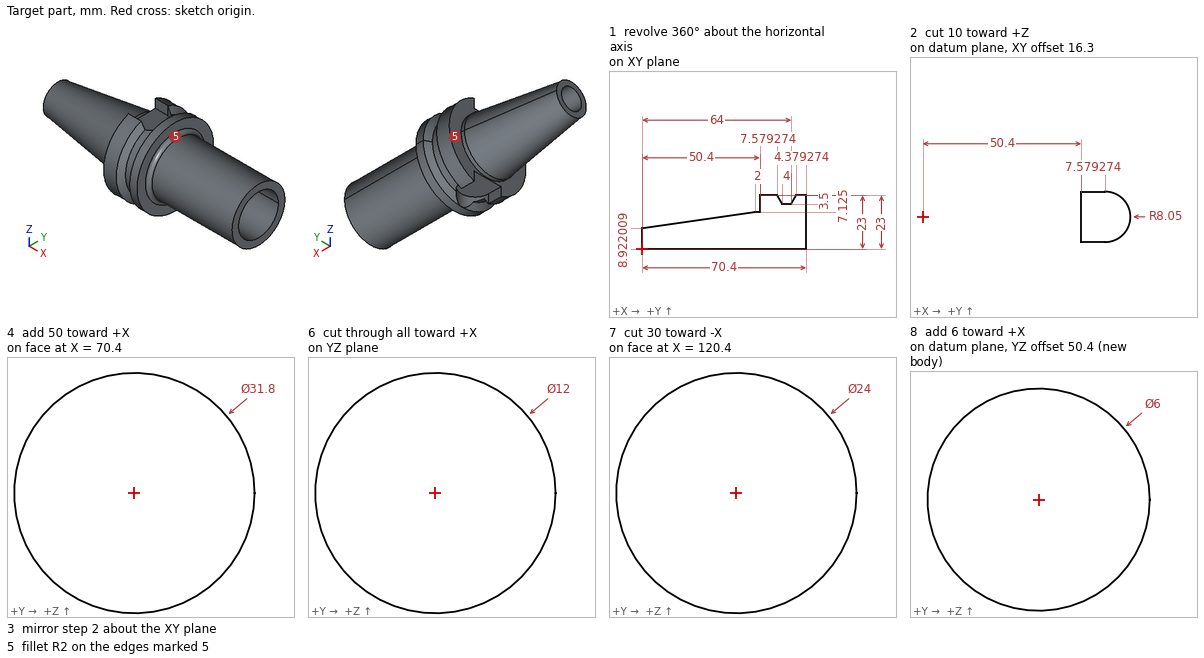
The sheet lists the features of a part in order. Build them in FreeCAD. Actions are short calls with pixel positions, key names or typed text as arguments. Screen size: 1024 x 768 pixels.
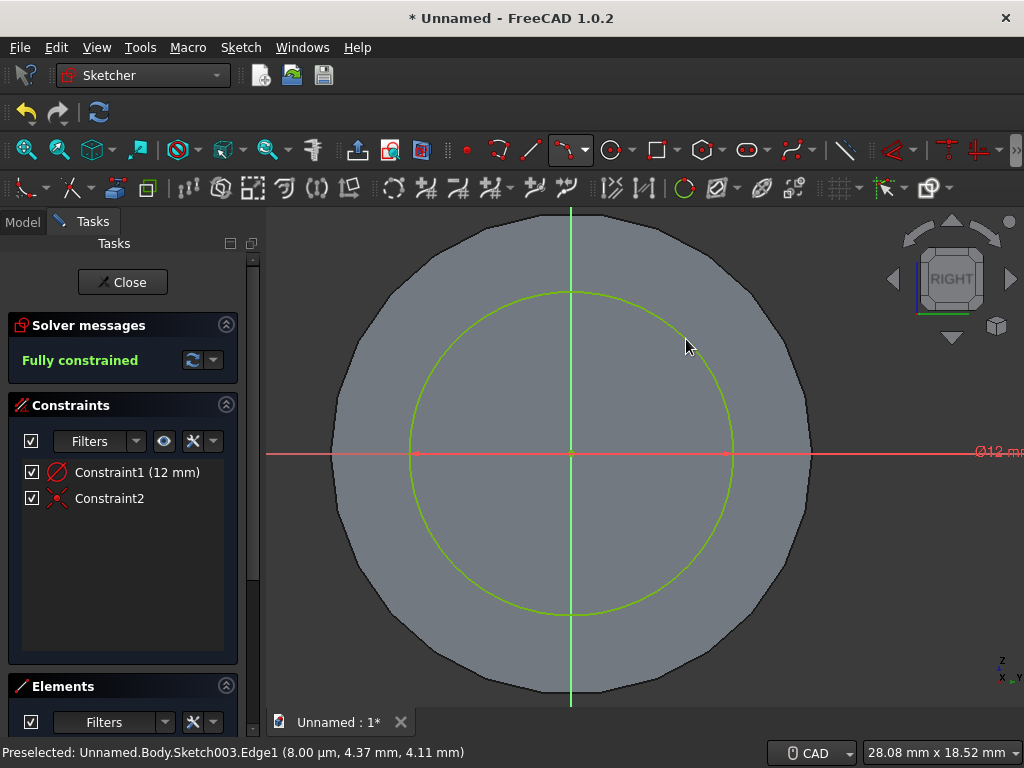
click(123, 282)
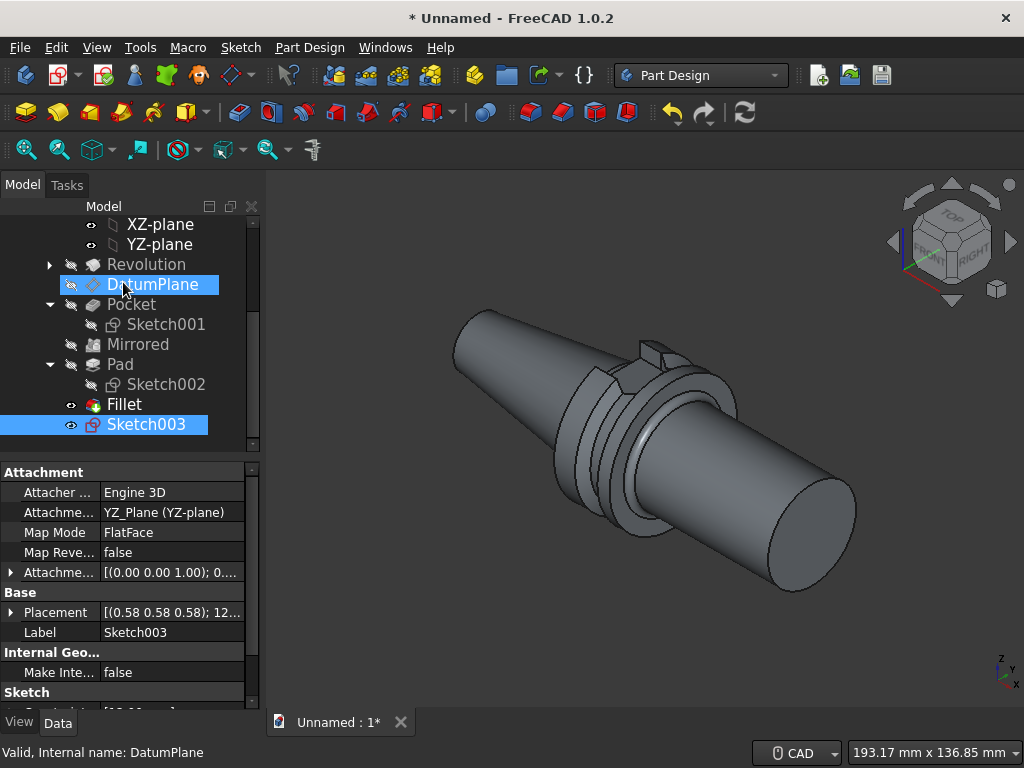
click(240, 112)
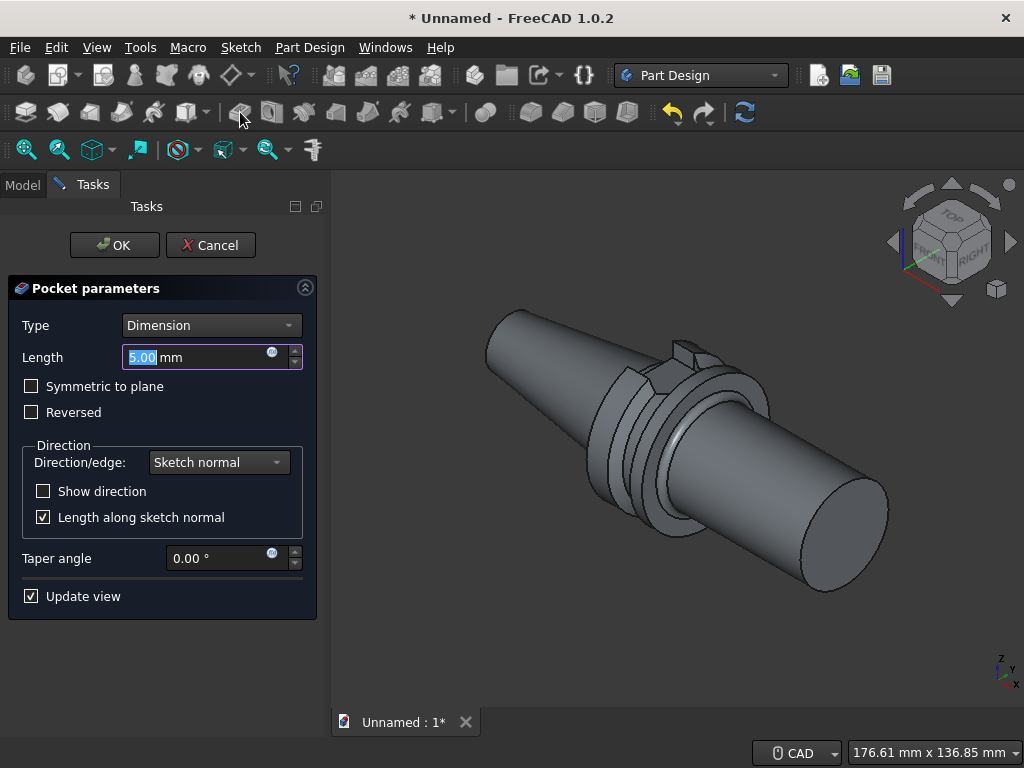
click(212, 326)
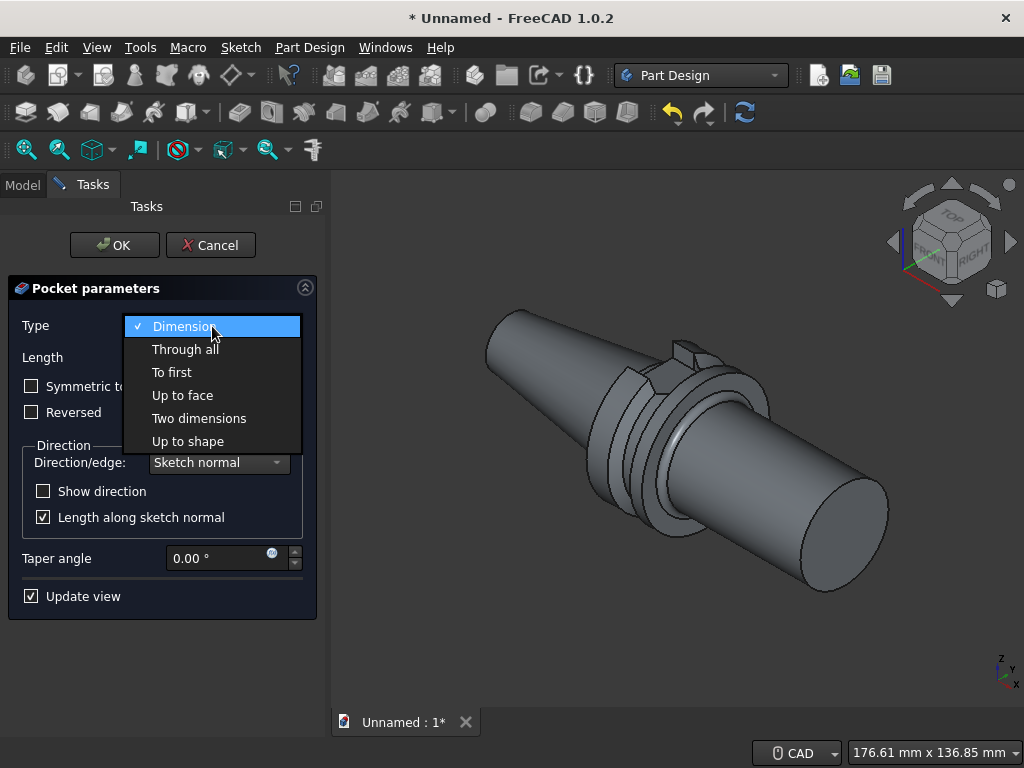
click(212, 350)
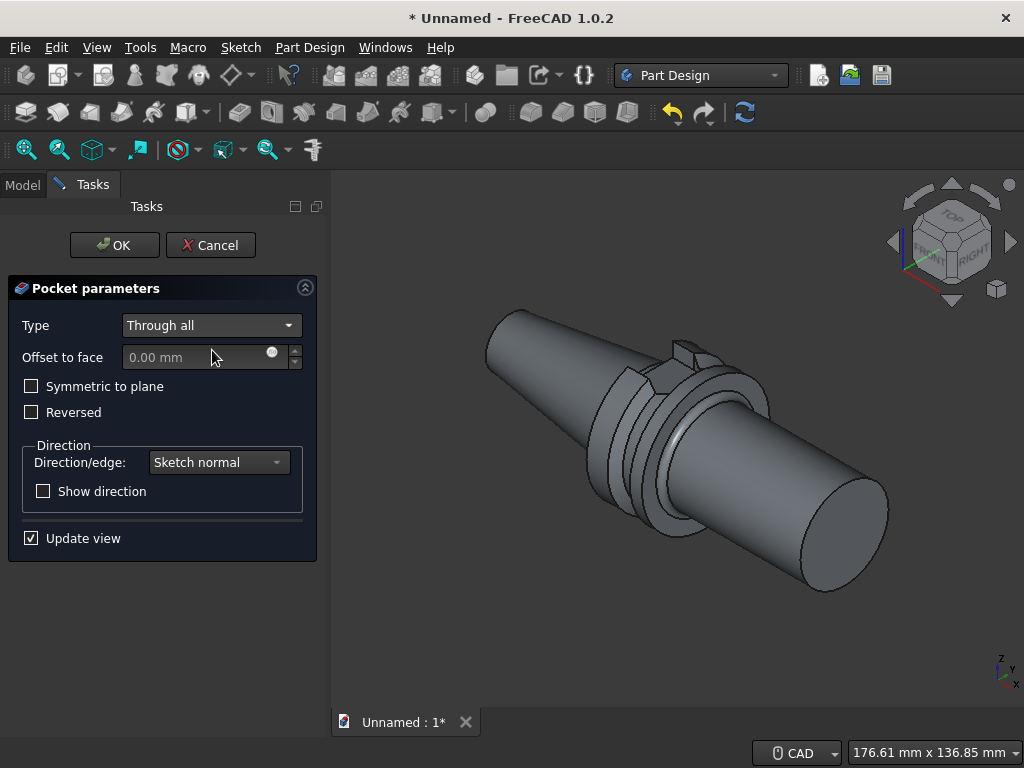
click(30, 412)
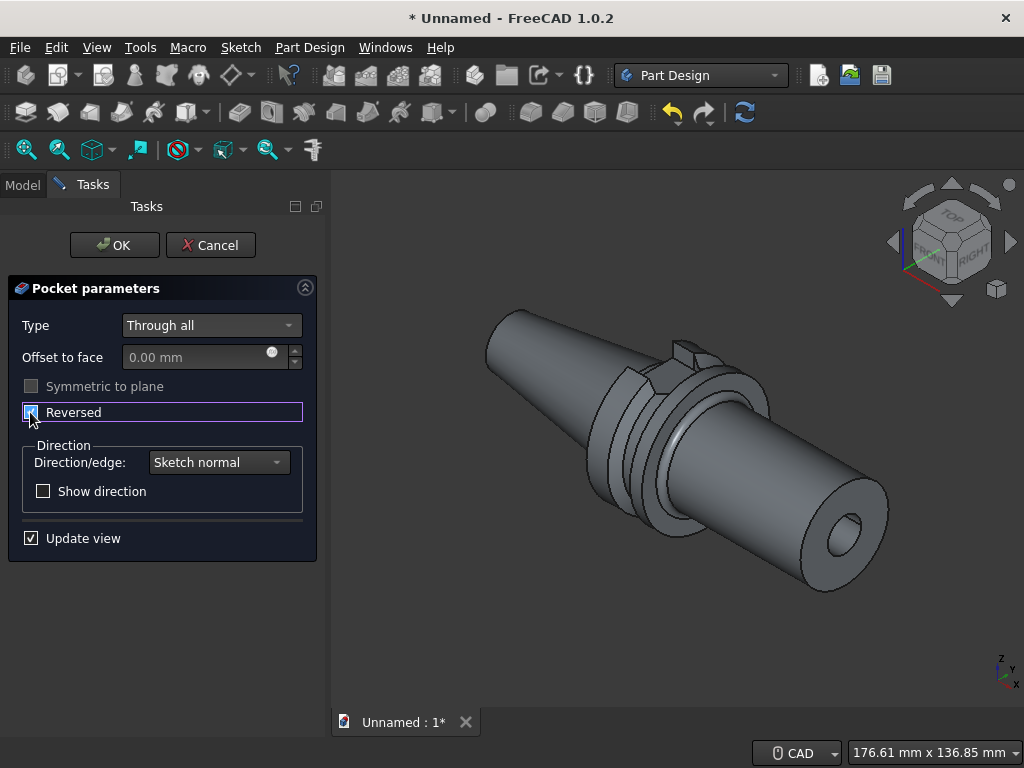
click(115, 245)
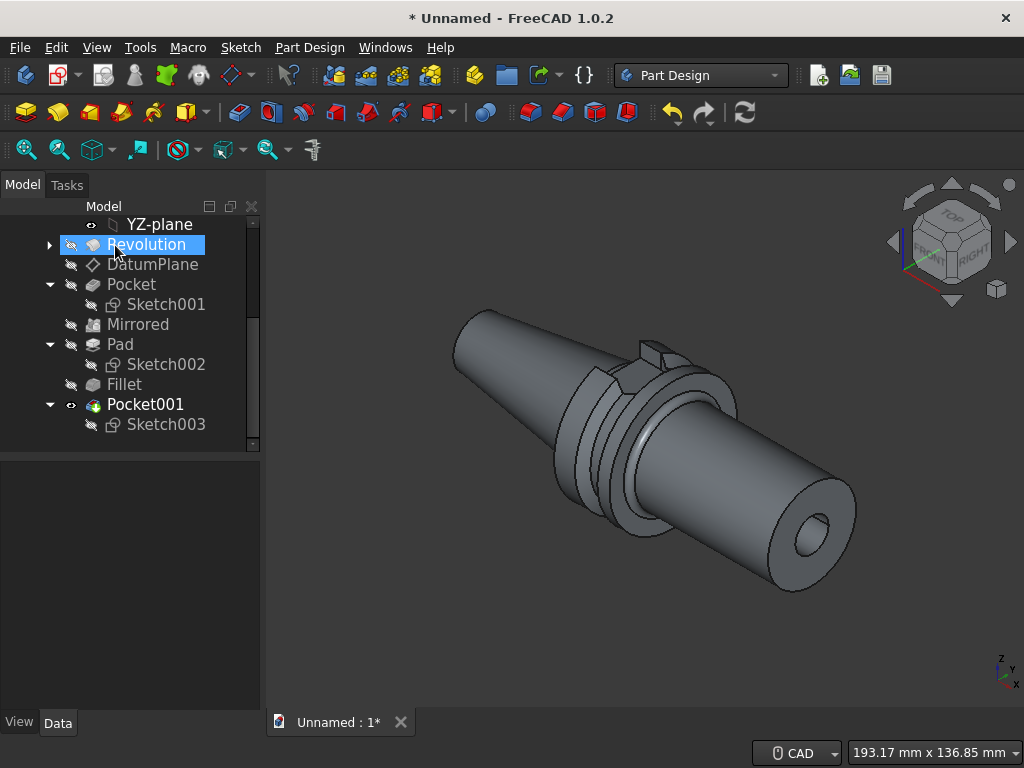
click(825, 498)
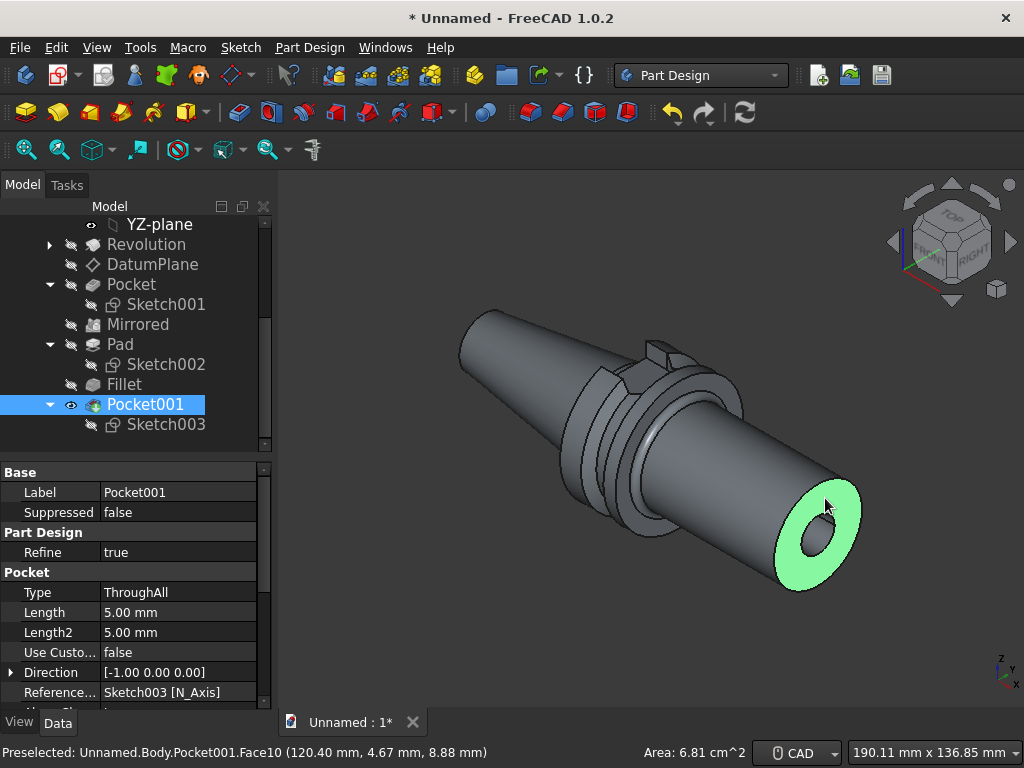
click(58, 76)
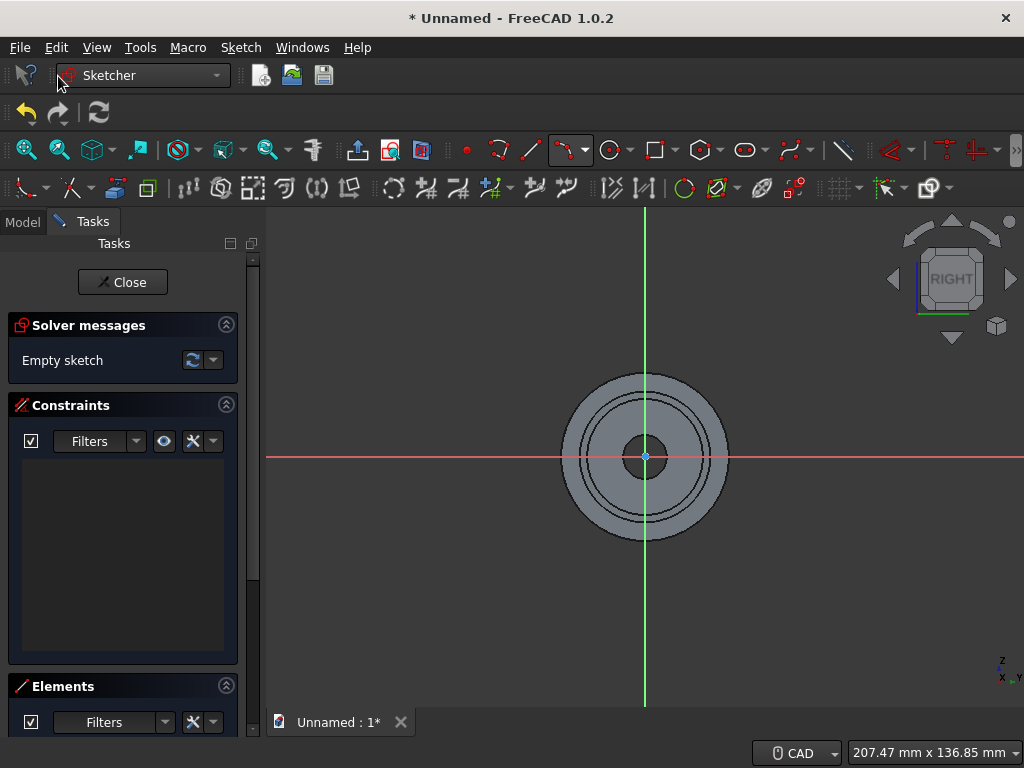
scroll(675, 457, up, 6)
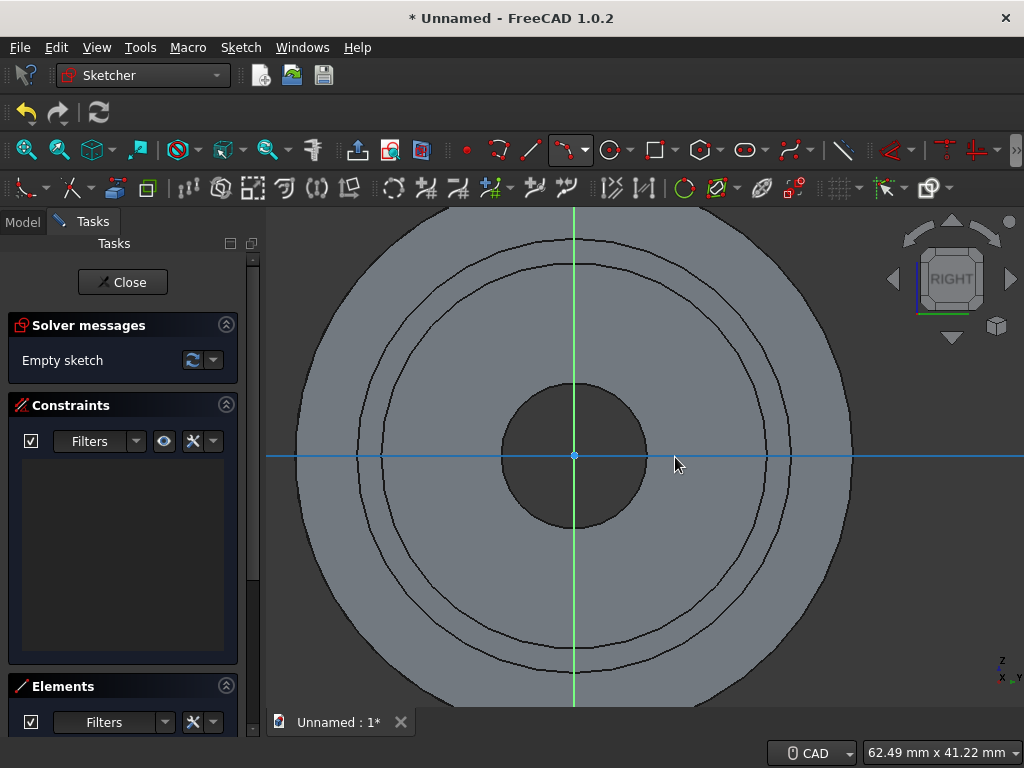
key(g)
key(c)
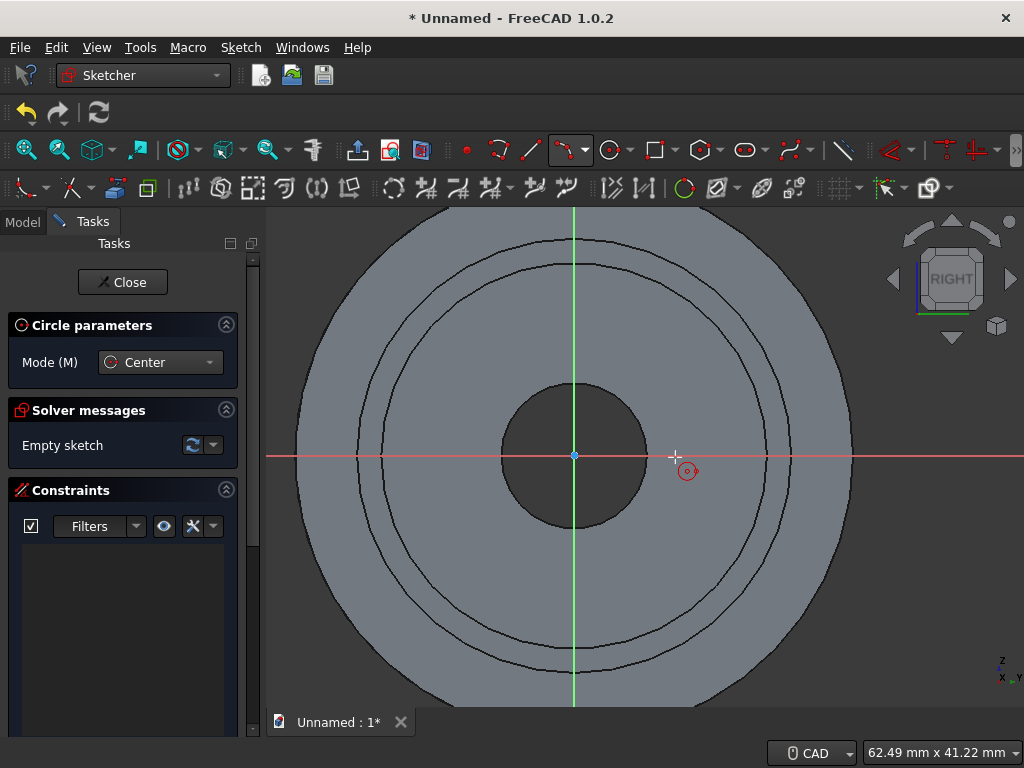
click(574, 456)
move(677, 353)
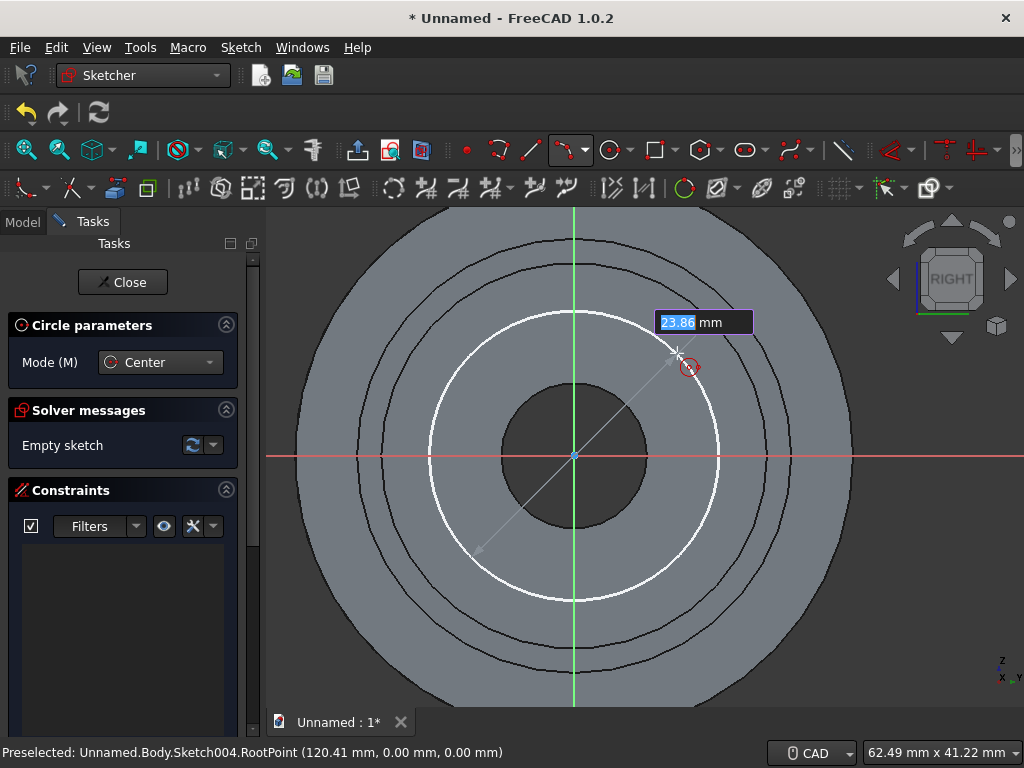
text(24)
key(Return)
key(Escape)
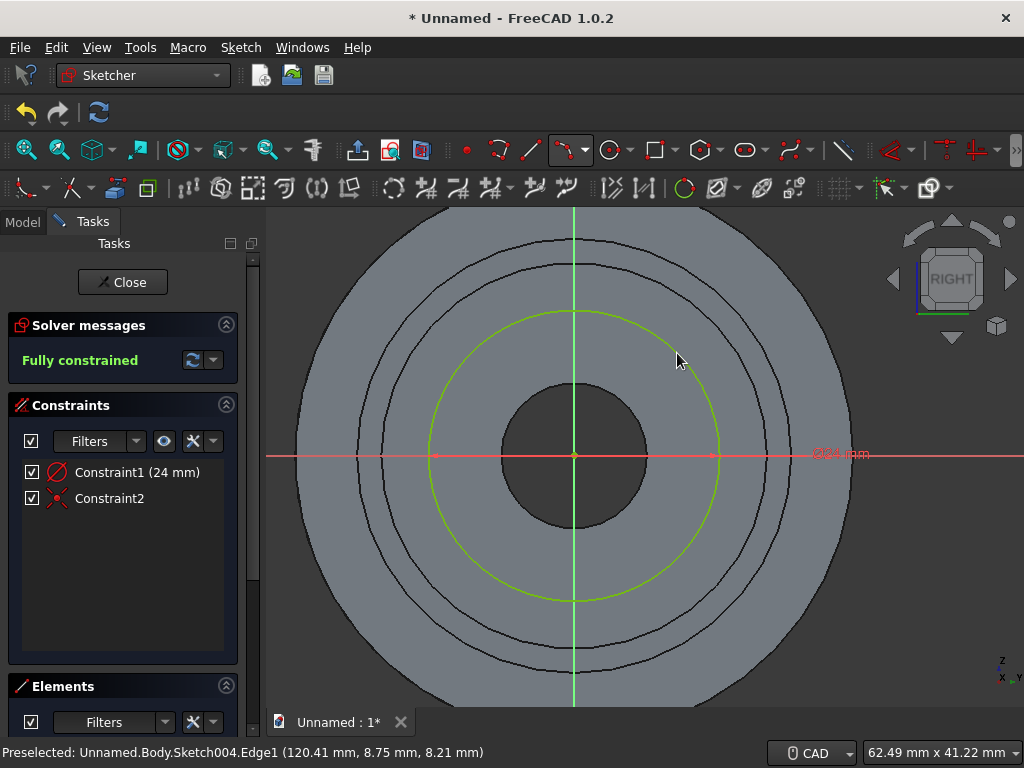
click(123, 282)